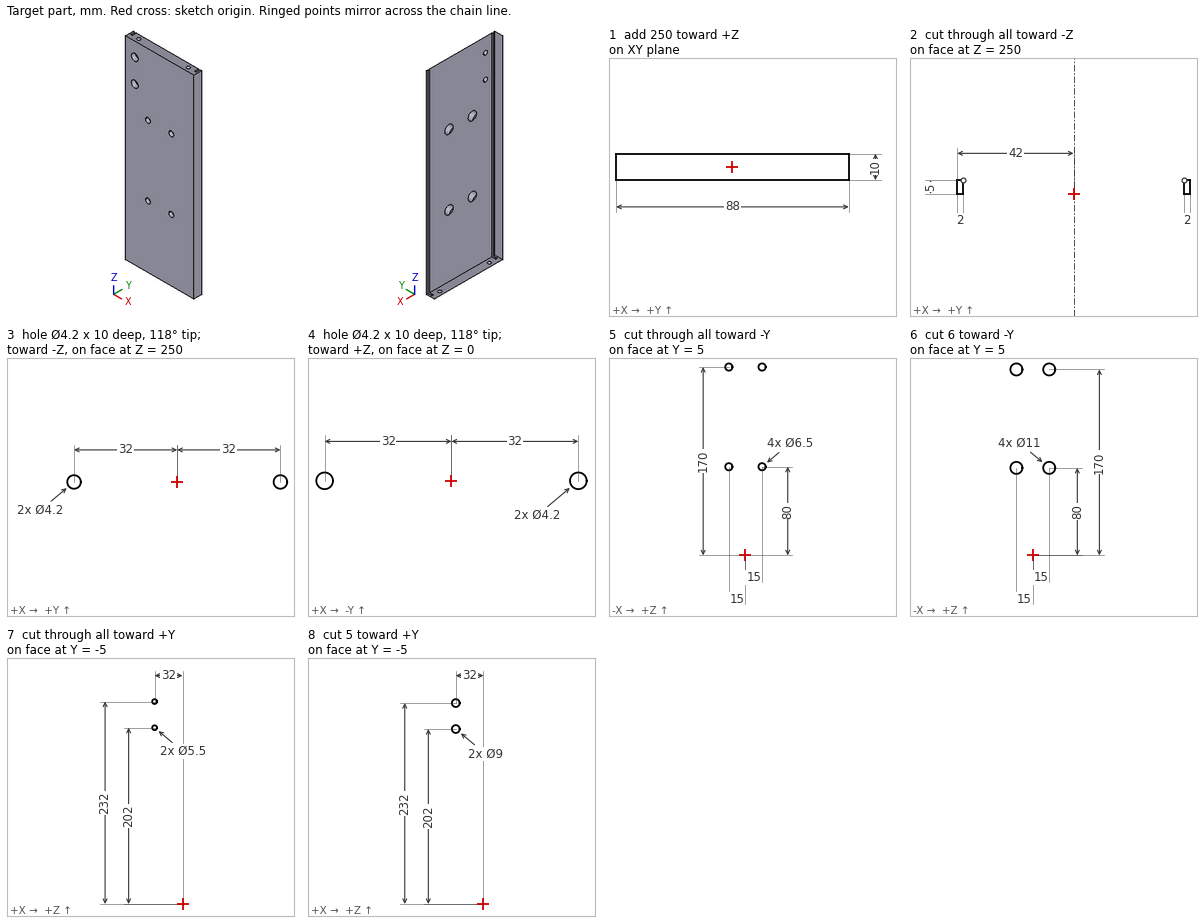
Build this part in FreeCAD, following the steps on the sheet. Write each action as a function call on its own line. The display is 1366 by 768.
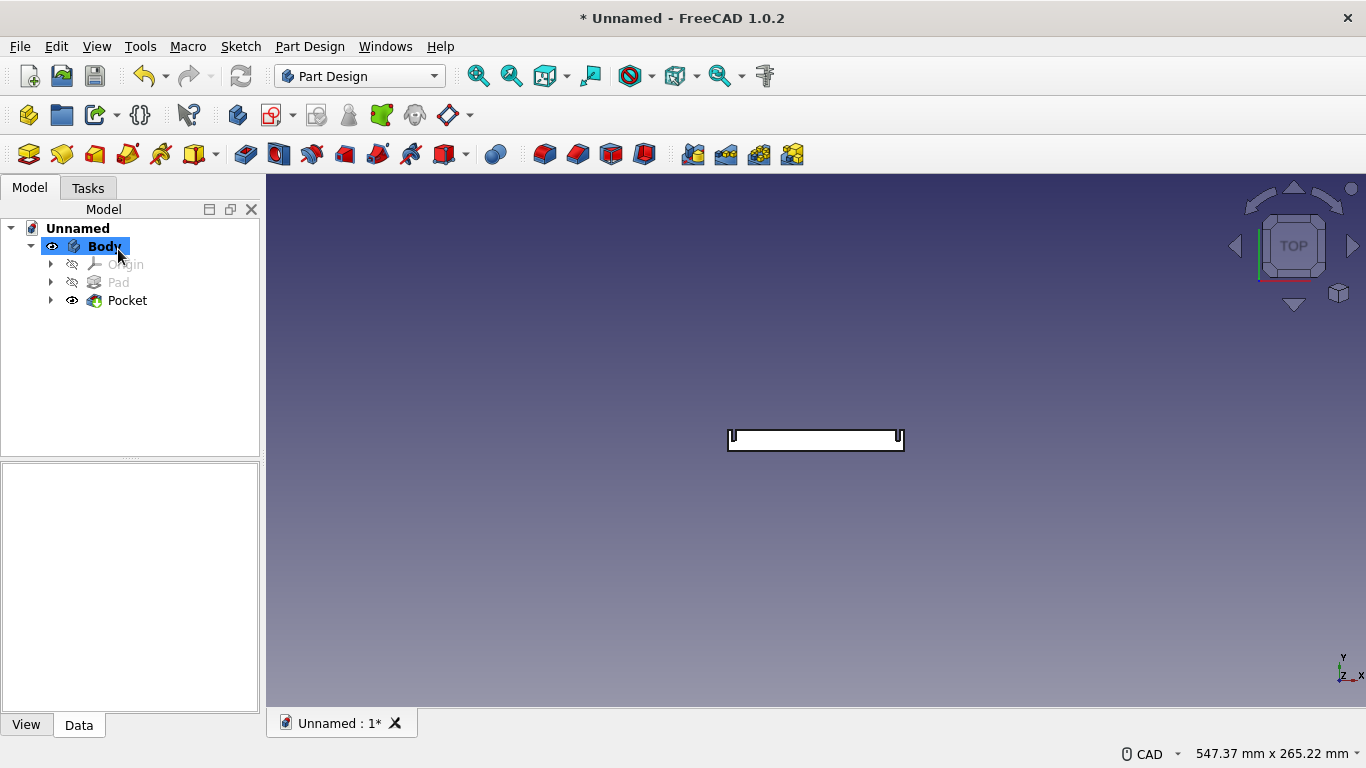
key(v)
key(f)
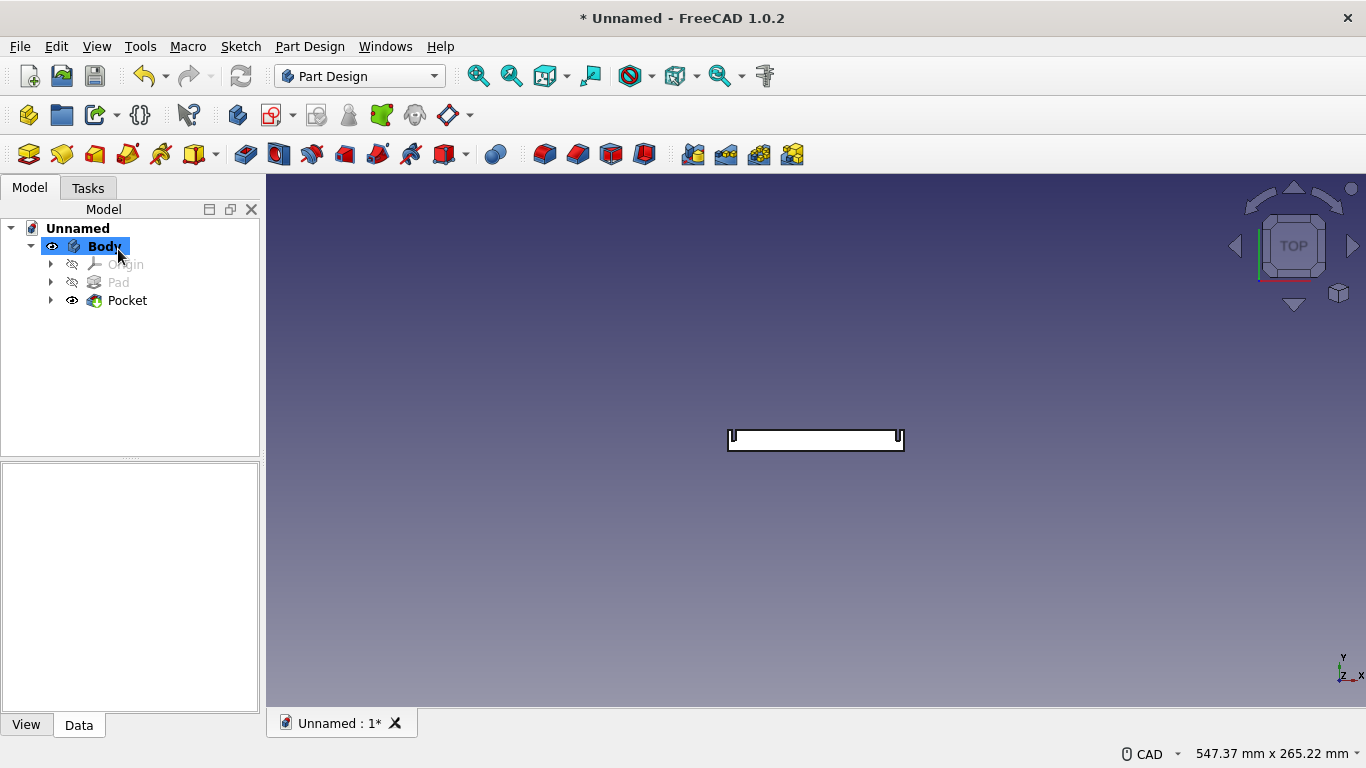
click(867, 439)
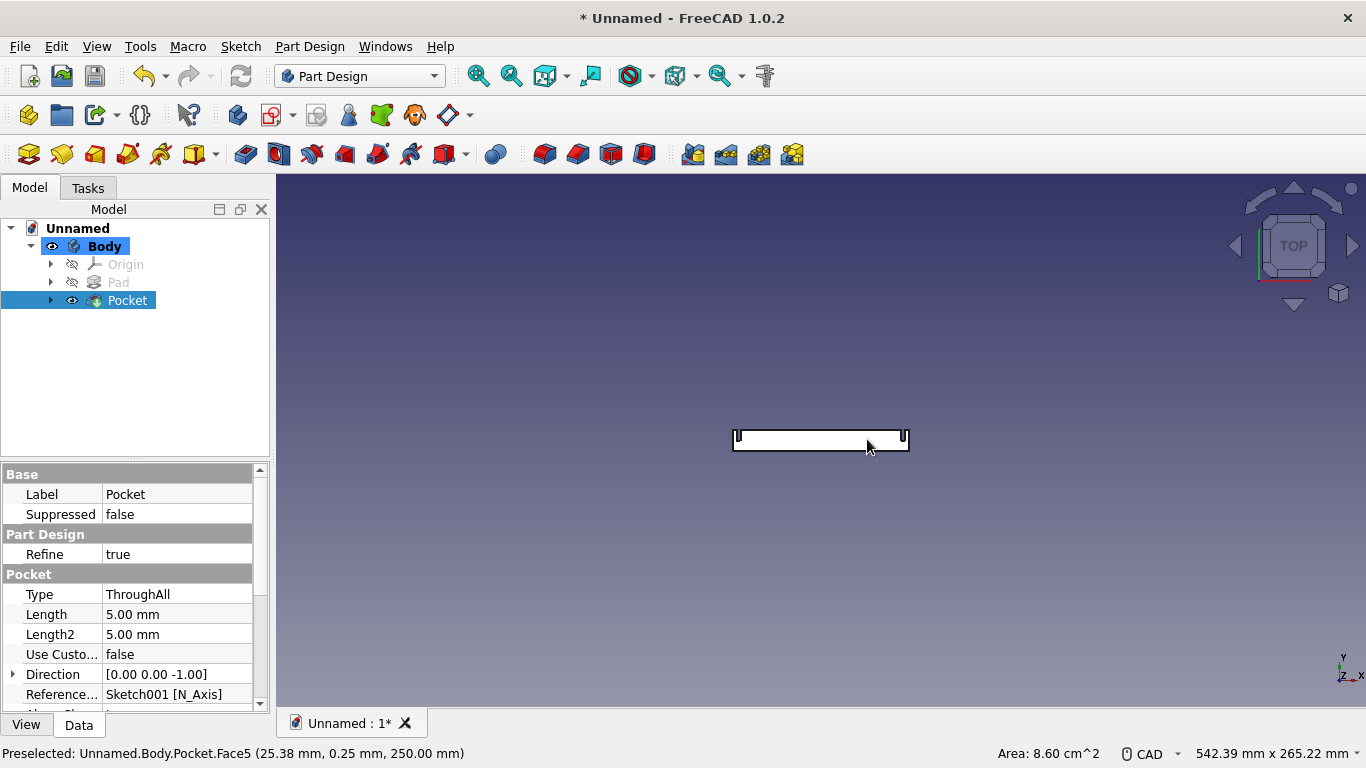
click(270, 116)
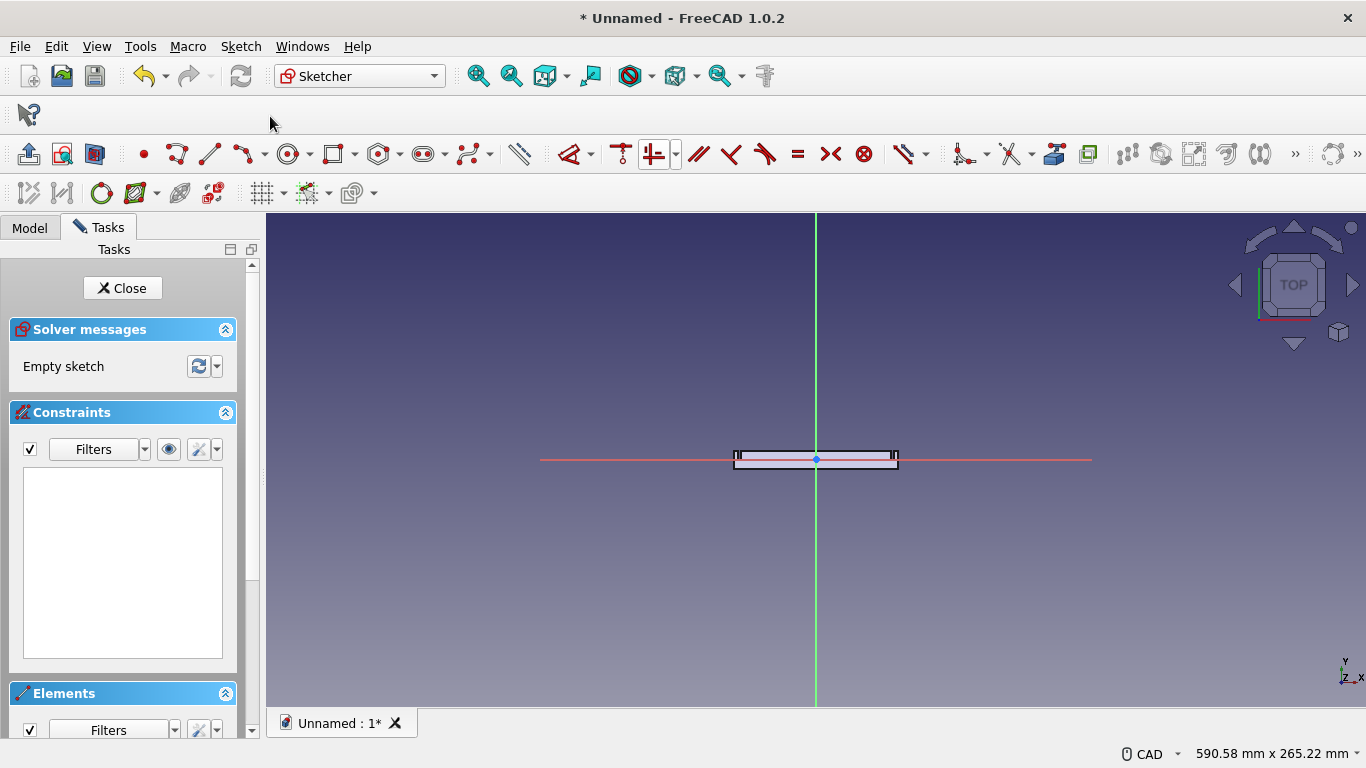
scroll(833, 460, up, 8)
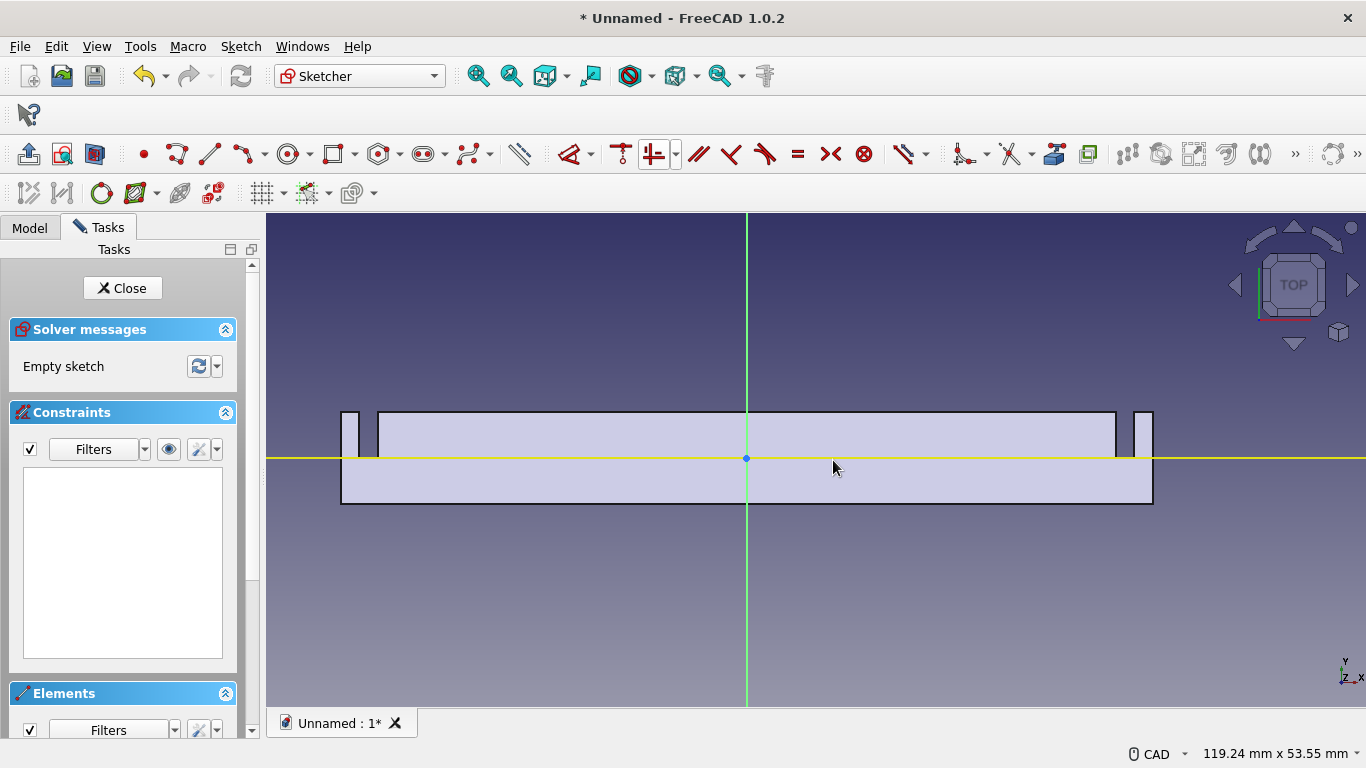
key(g)
key(c)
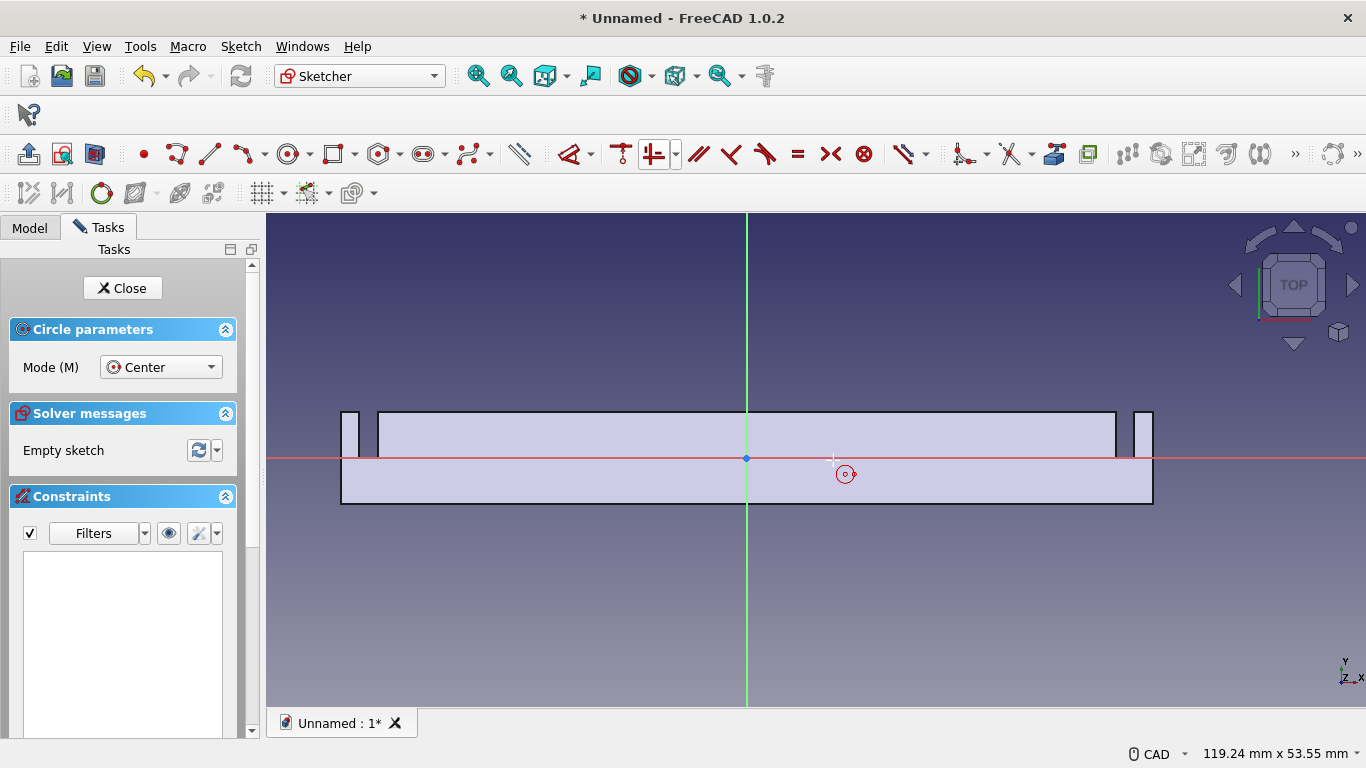
click(452, 458)
move(458, 440)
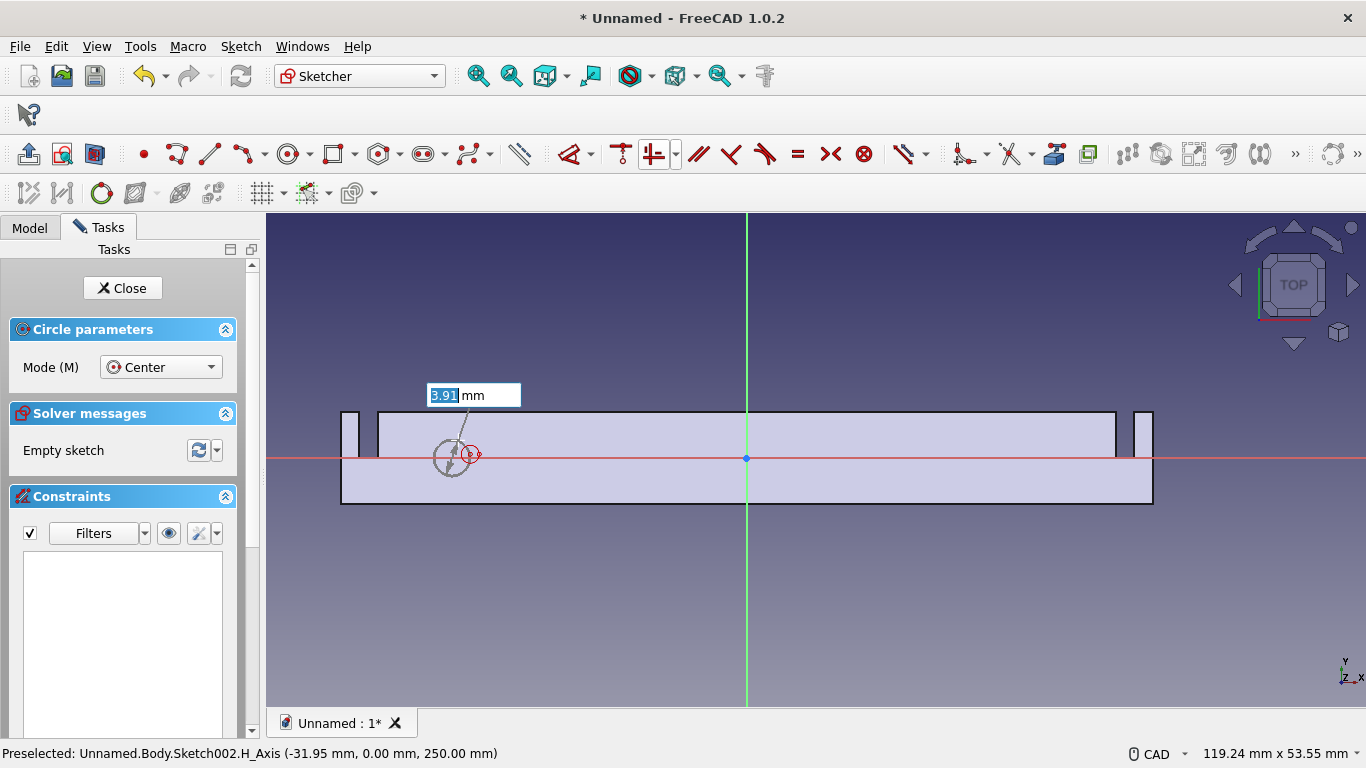
text(4.2)
key(Return)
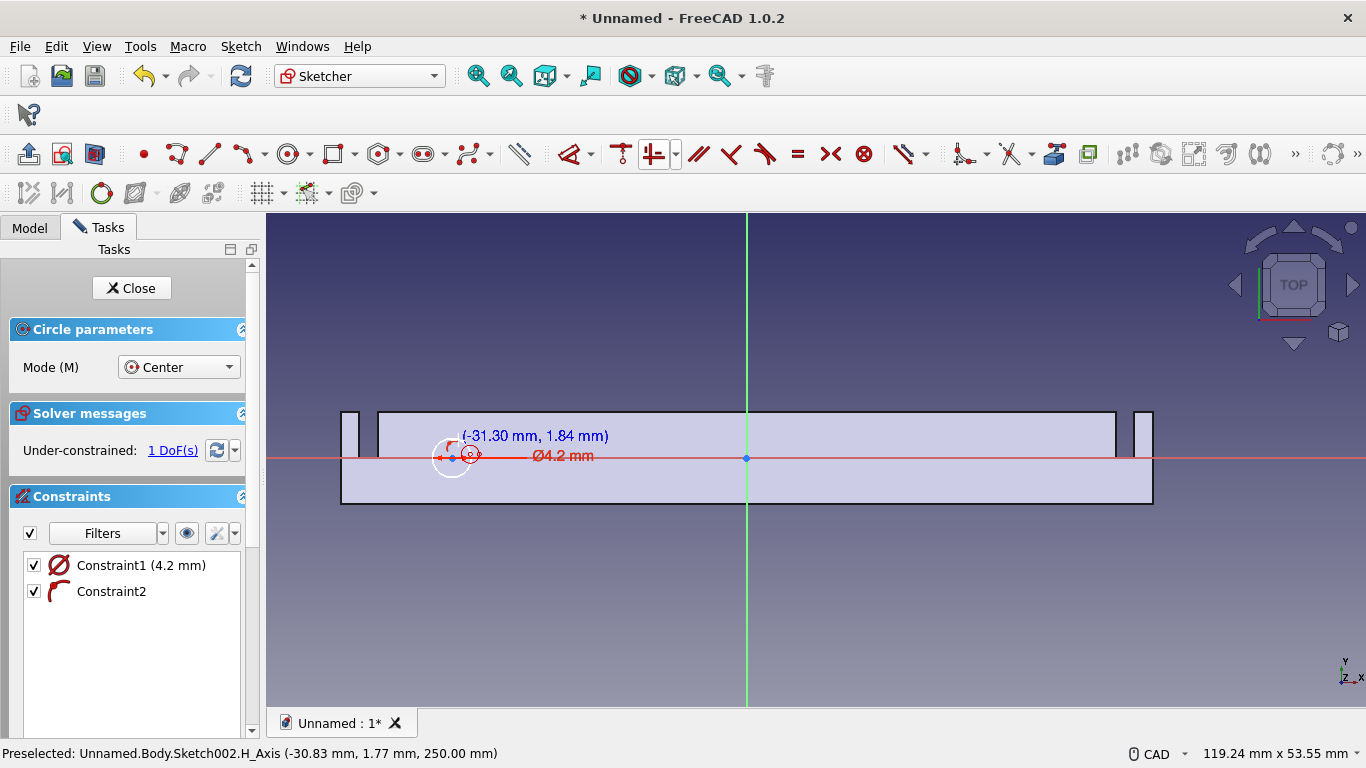
click(1042, 458)
move(1049, 440)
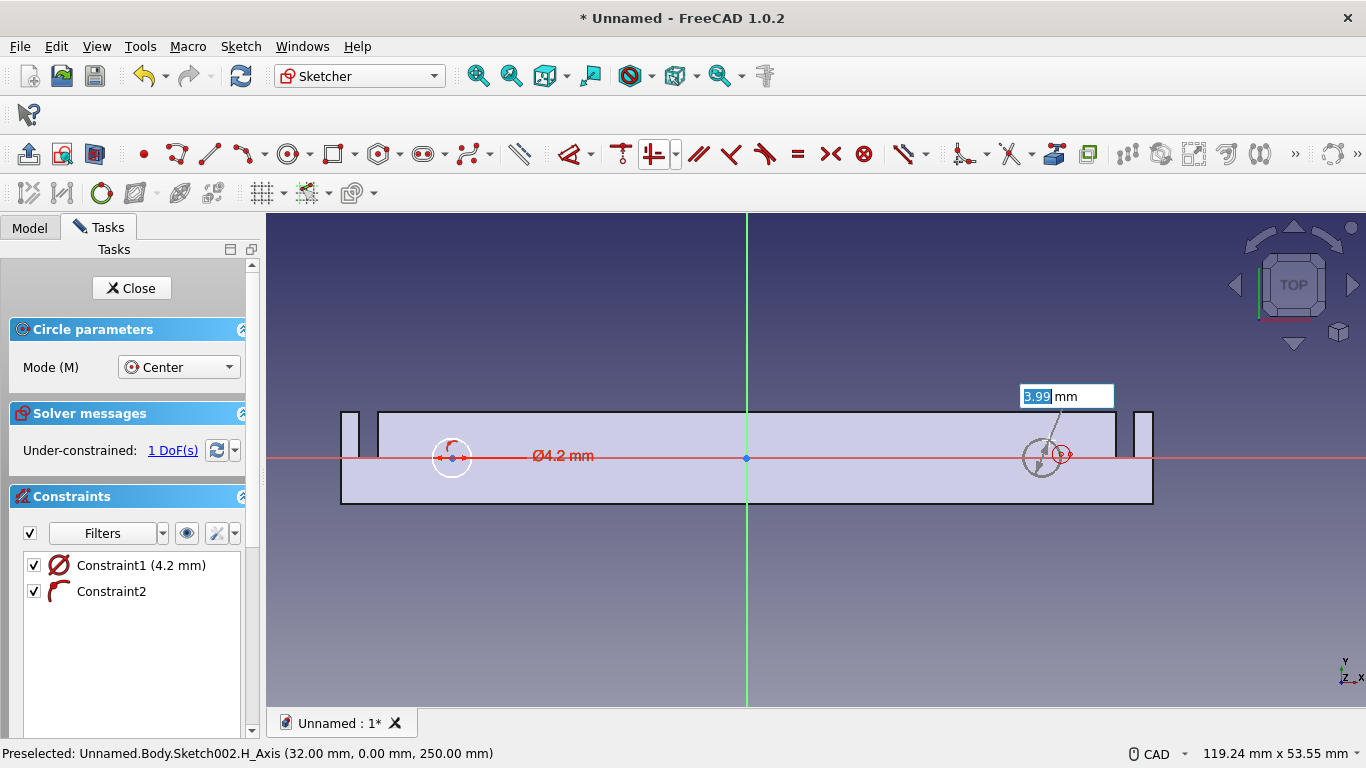
text(4.2)
key(Return)
key(Escape)